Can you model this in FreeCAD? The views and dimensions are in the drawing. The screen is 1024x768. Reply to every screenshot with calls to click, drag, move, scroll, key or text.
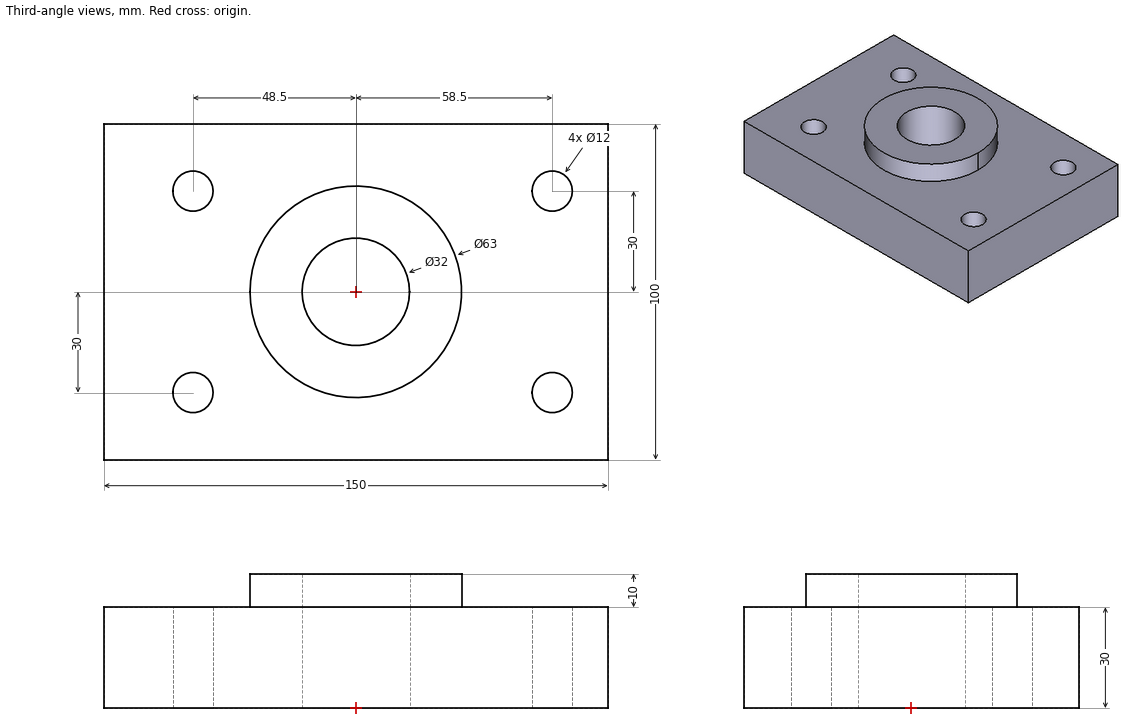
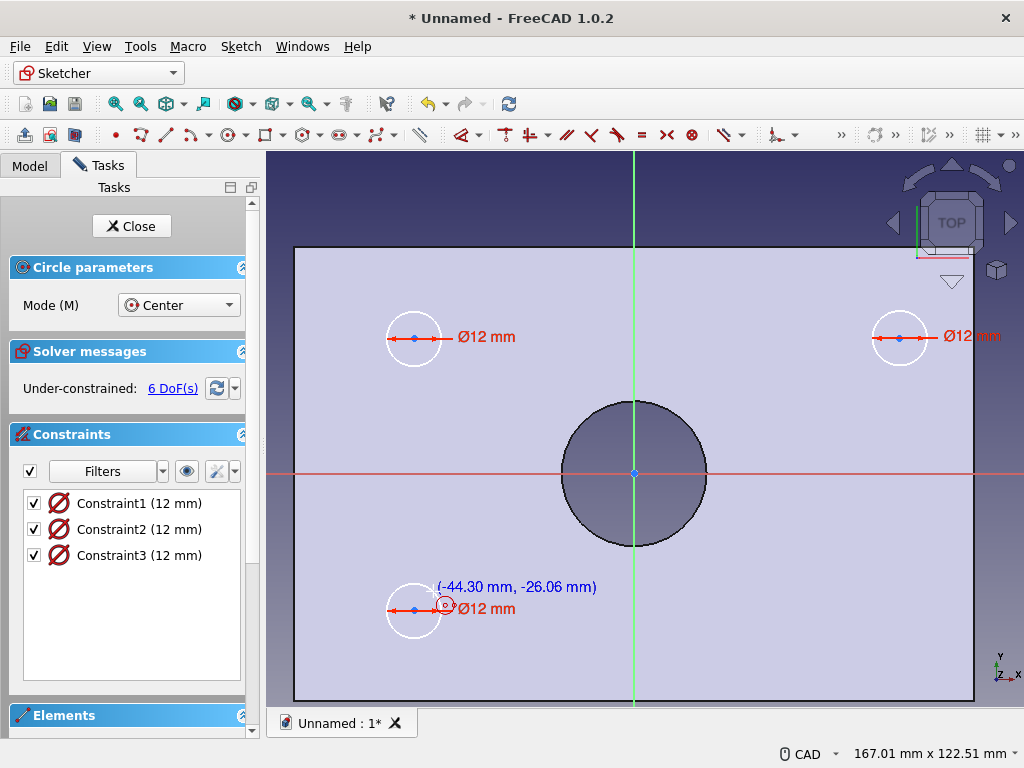
scroll(413, 338, down, 2)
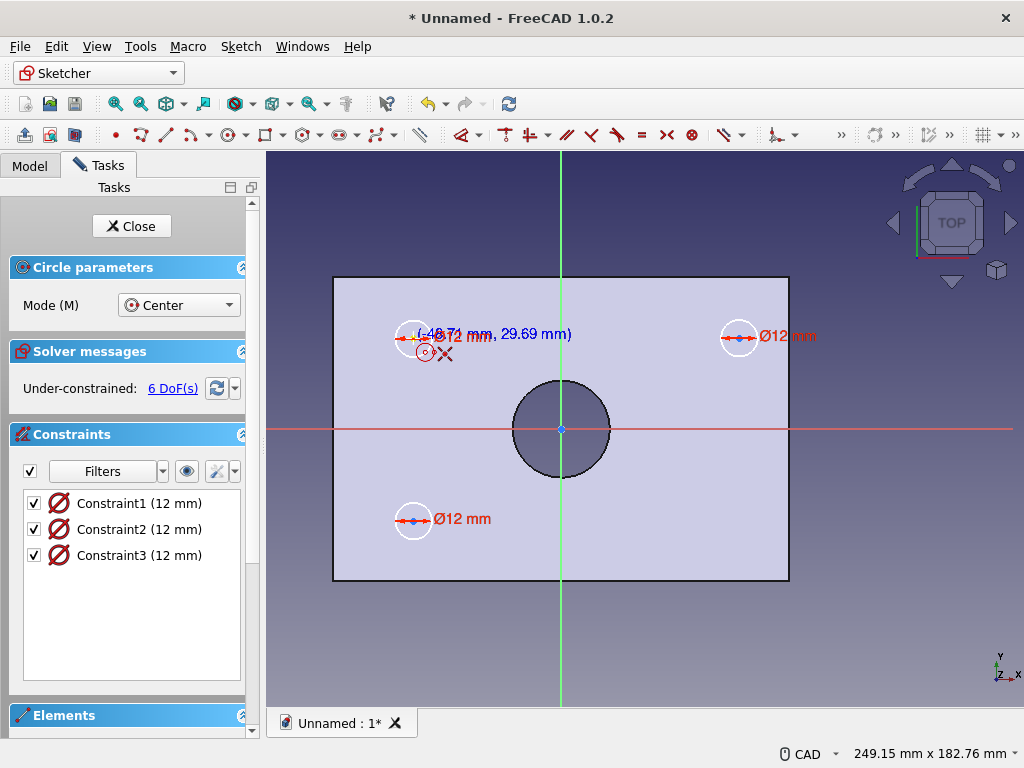
scroll(739, 520, up, 2)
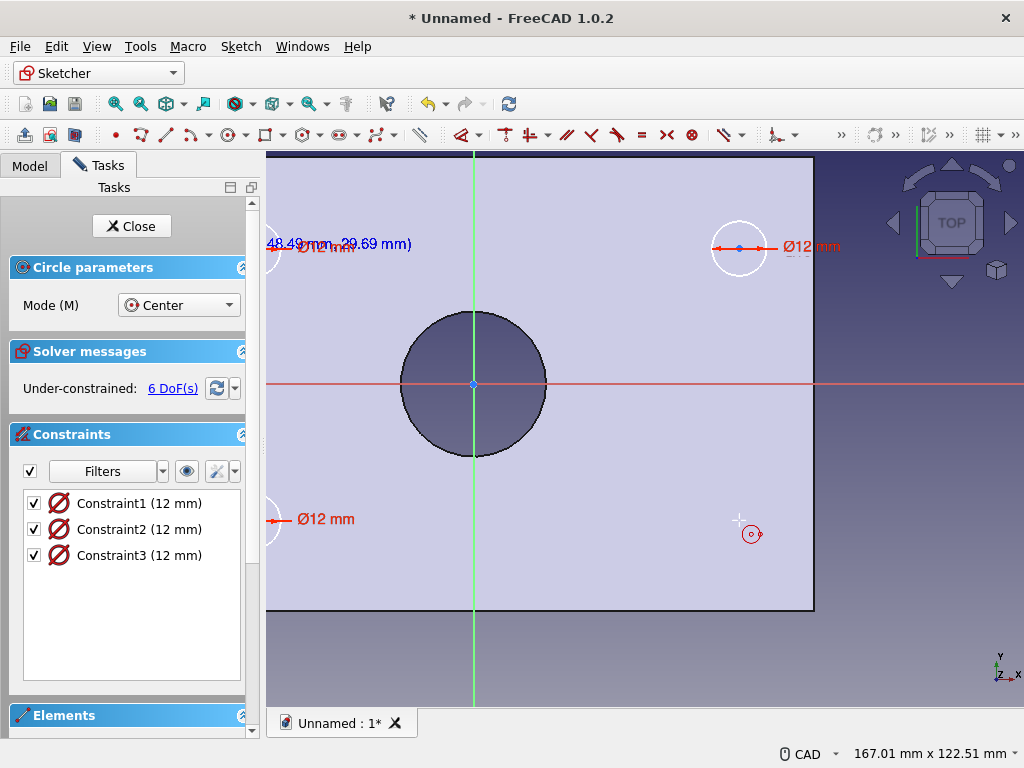
click(739, 520)
move(758, 501)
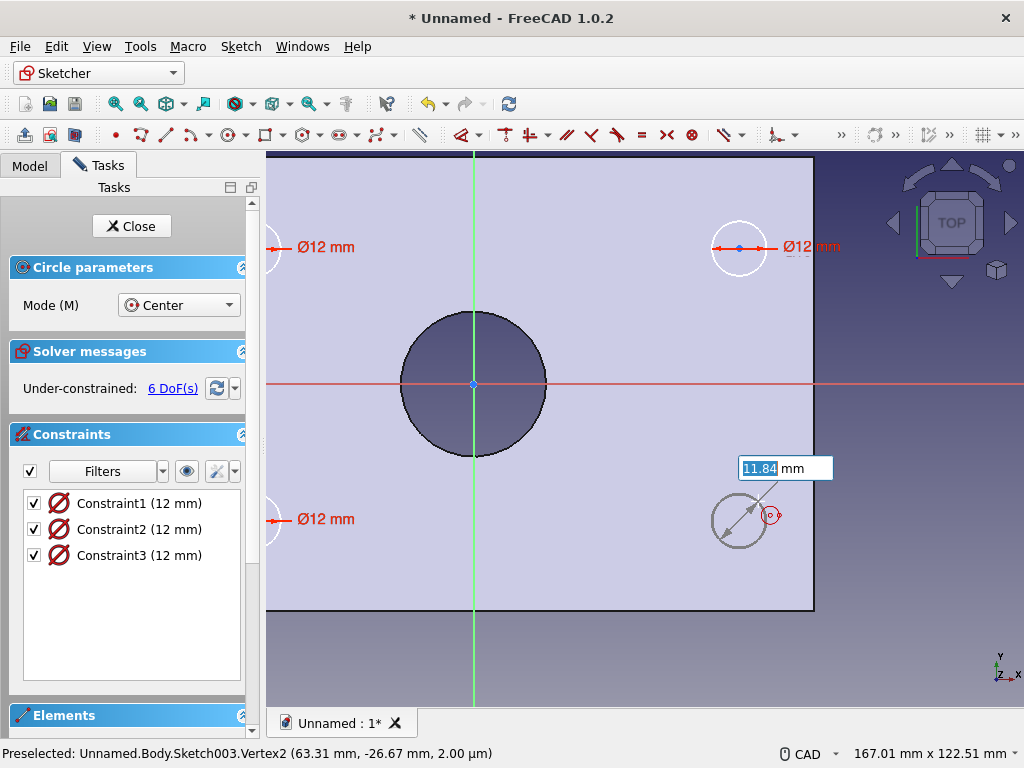
text(12)
key(Return)
key(Escape)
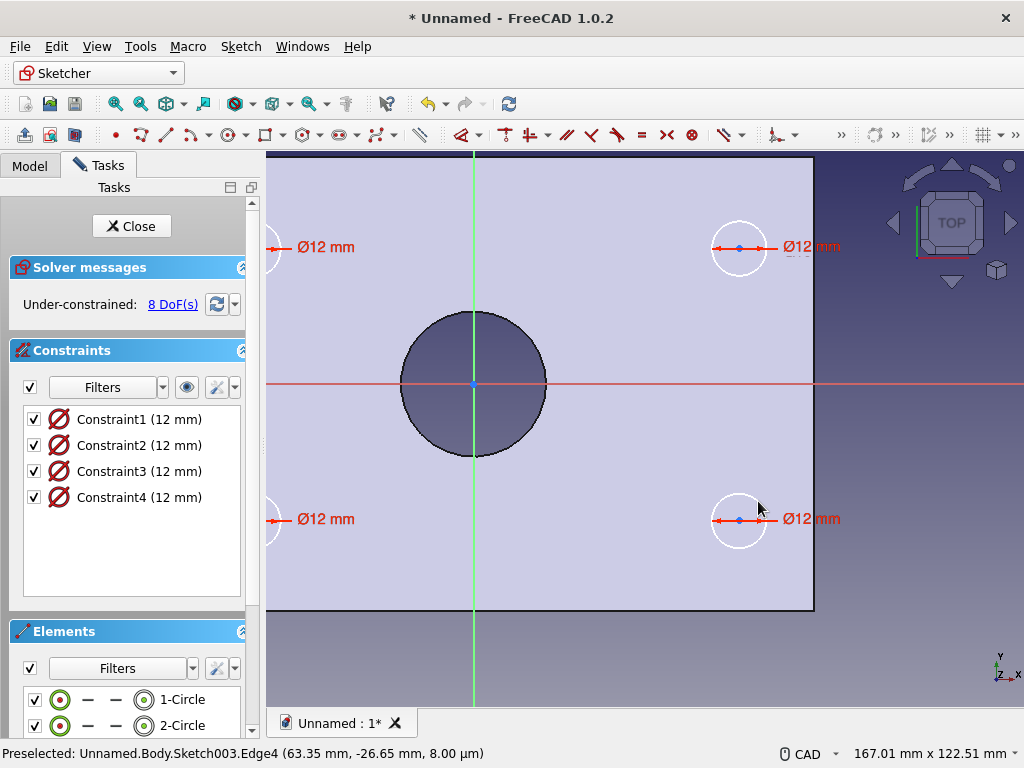
click(739, 249)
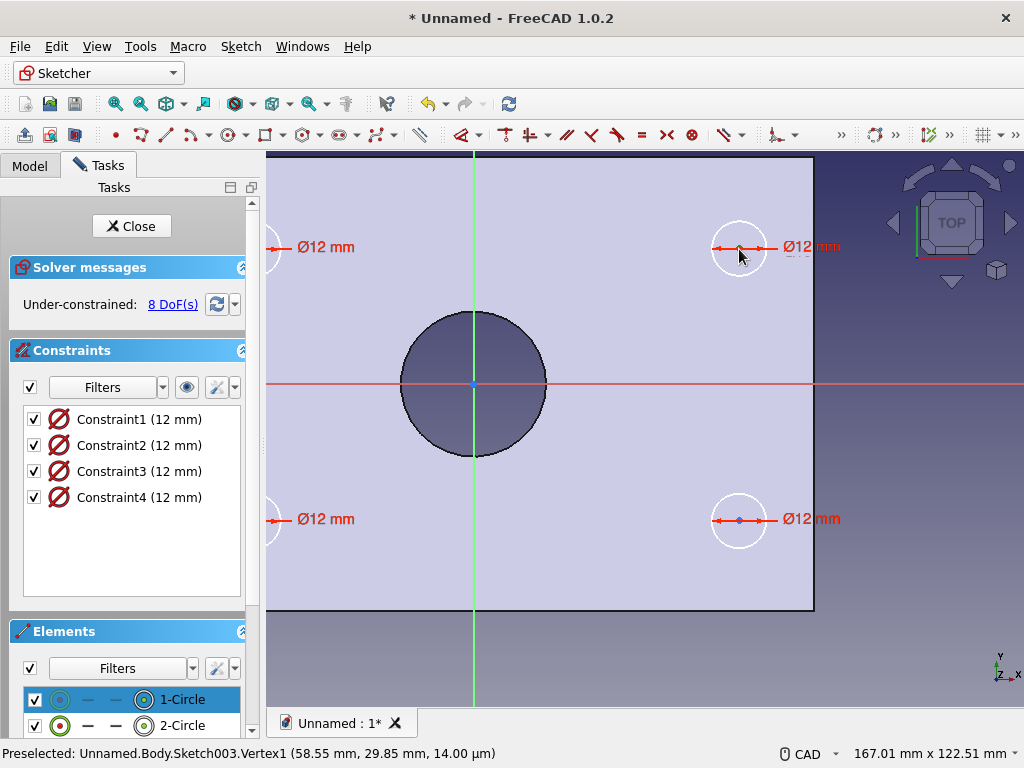
scroll(740, 520, down, 2)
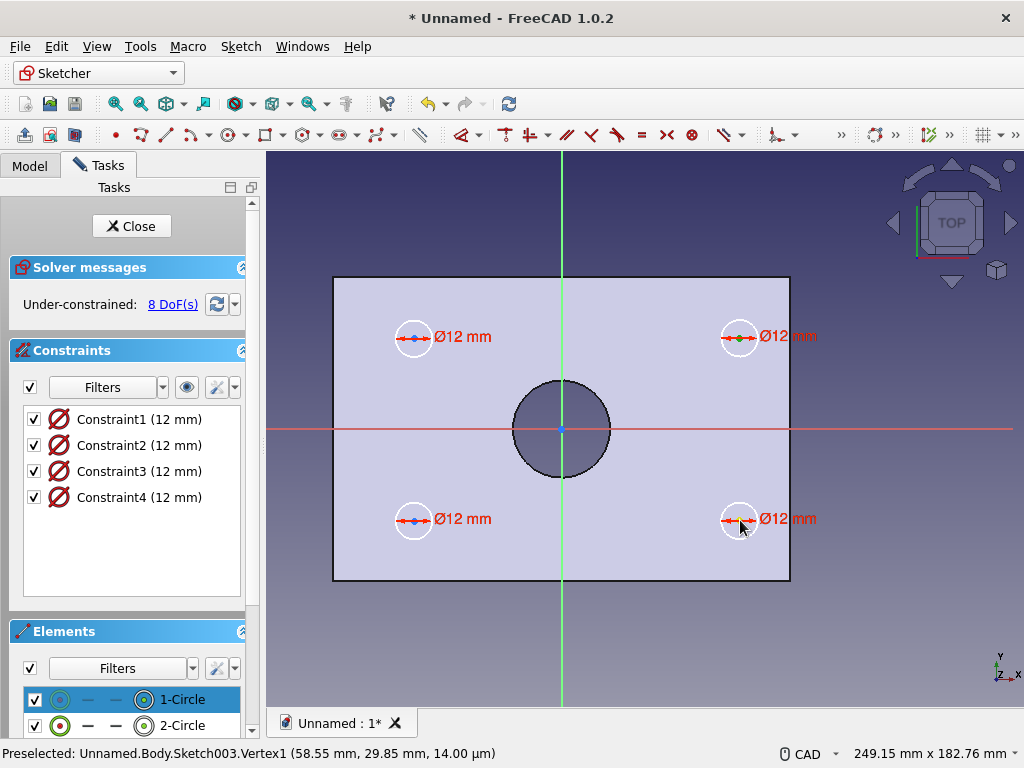
click(414, 339)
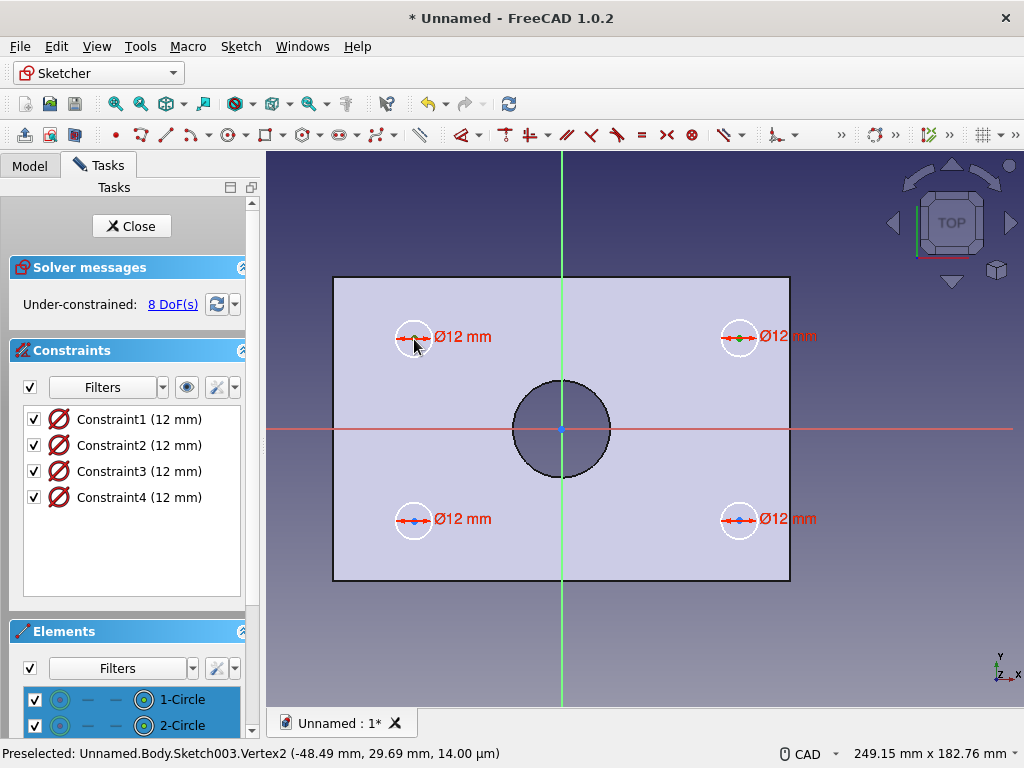
key(h)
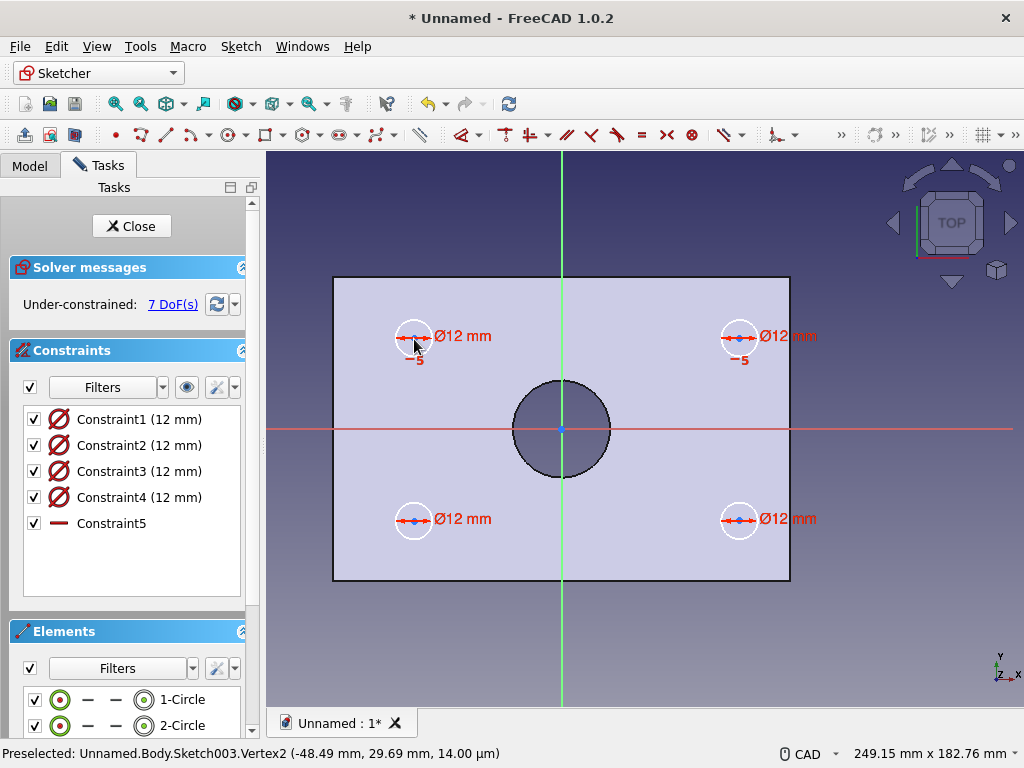
click(414, 338)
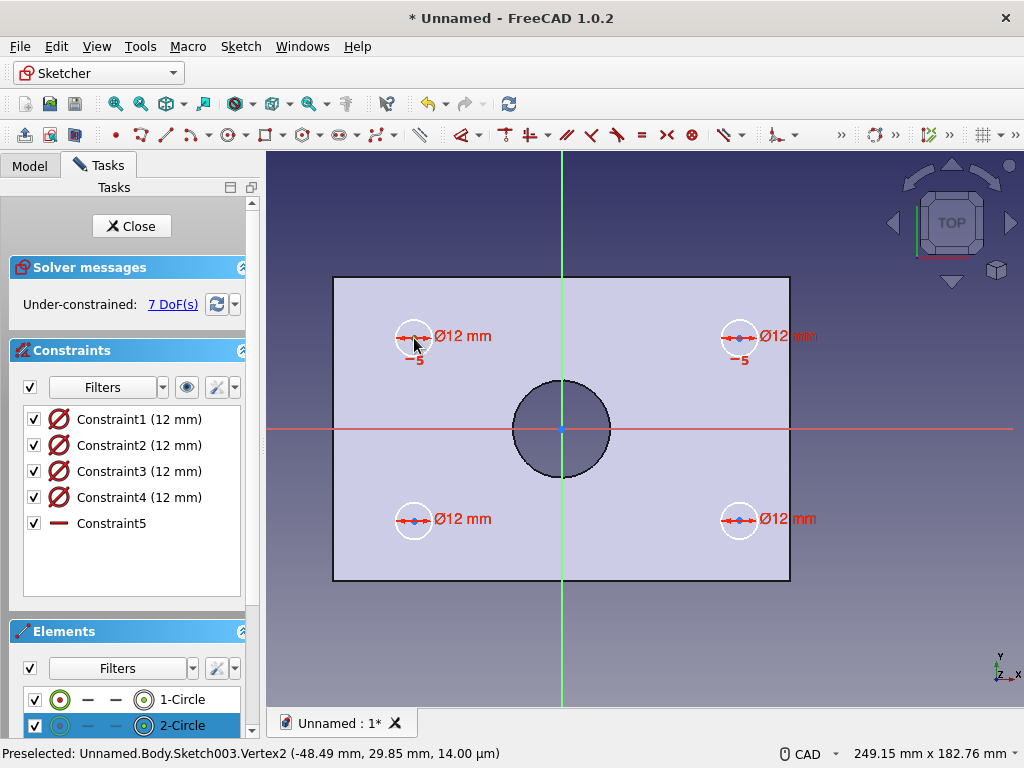
click(414, 521)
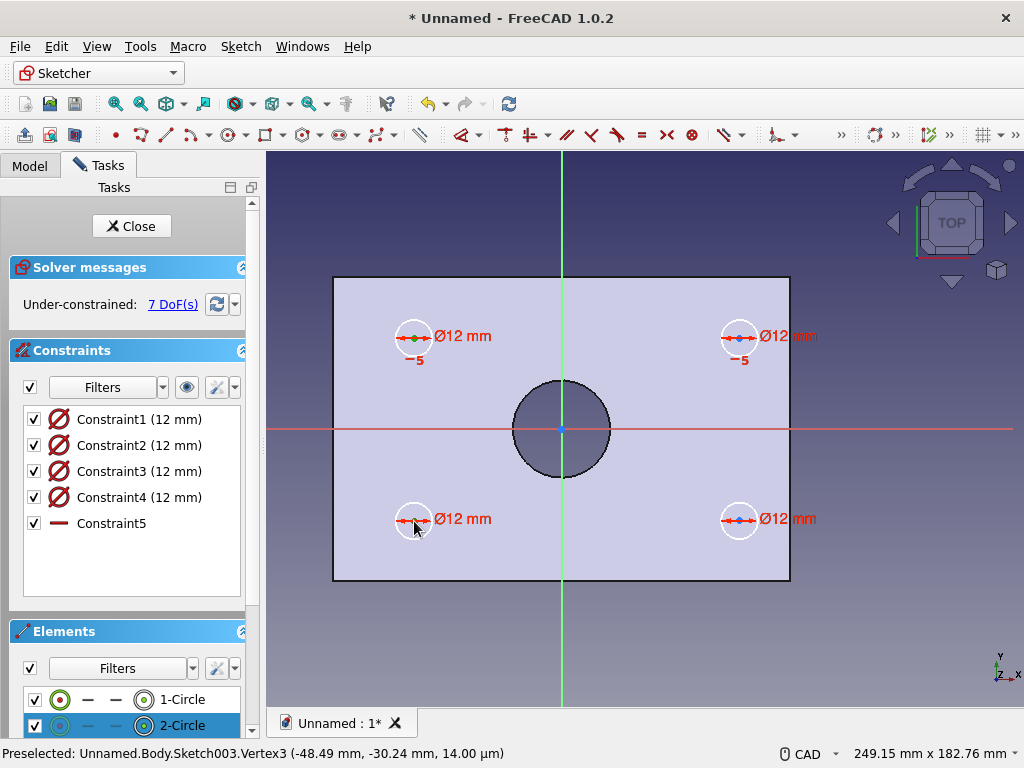
click(548, 136)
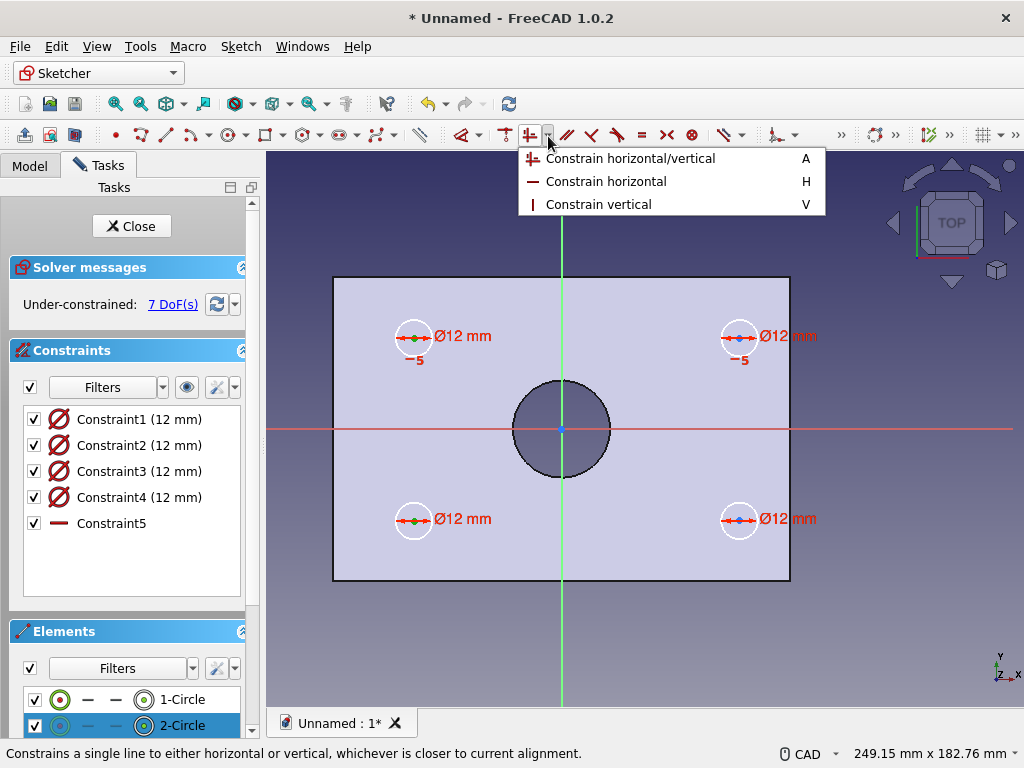
click(672, 204)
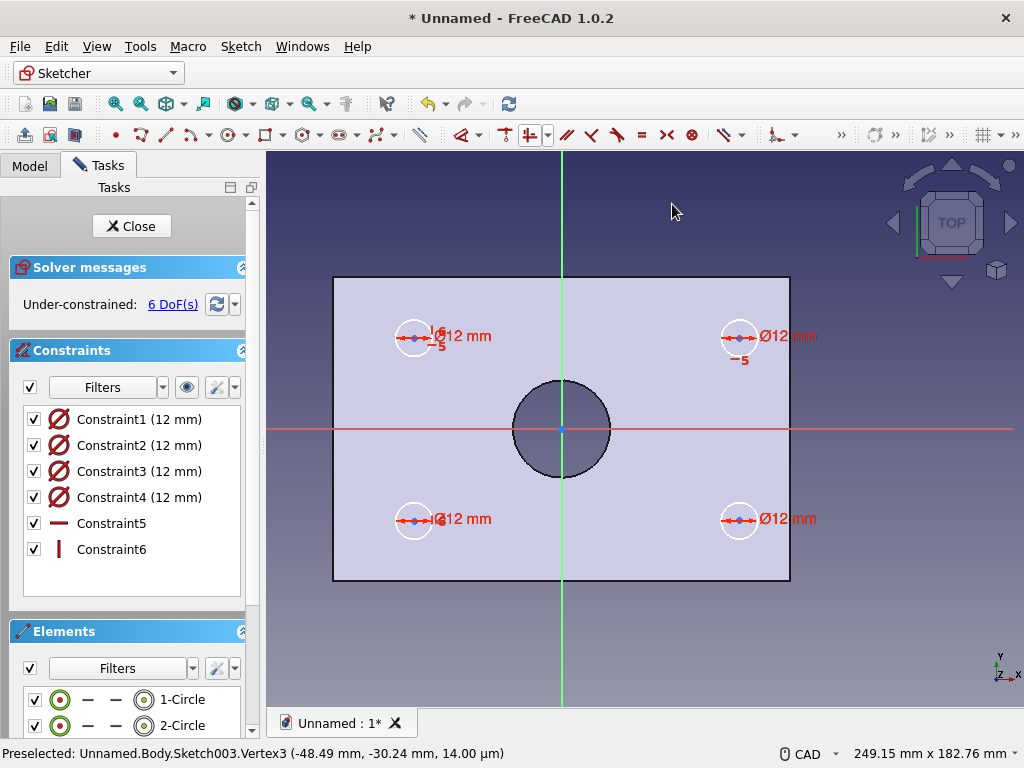
click(740, 338)